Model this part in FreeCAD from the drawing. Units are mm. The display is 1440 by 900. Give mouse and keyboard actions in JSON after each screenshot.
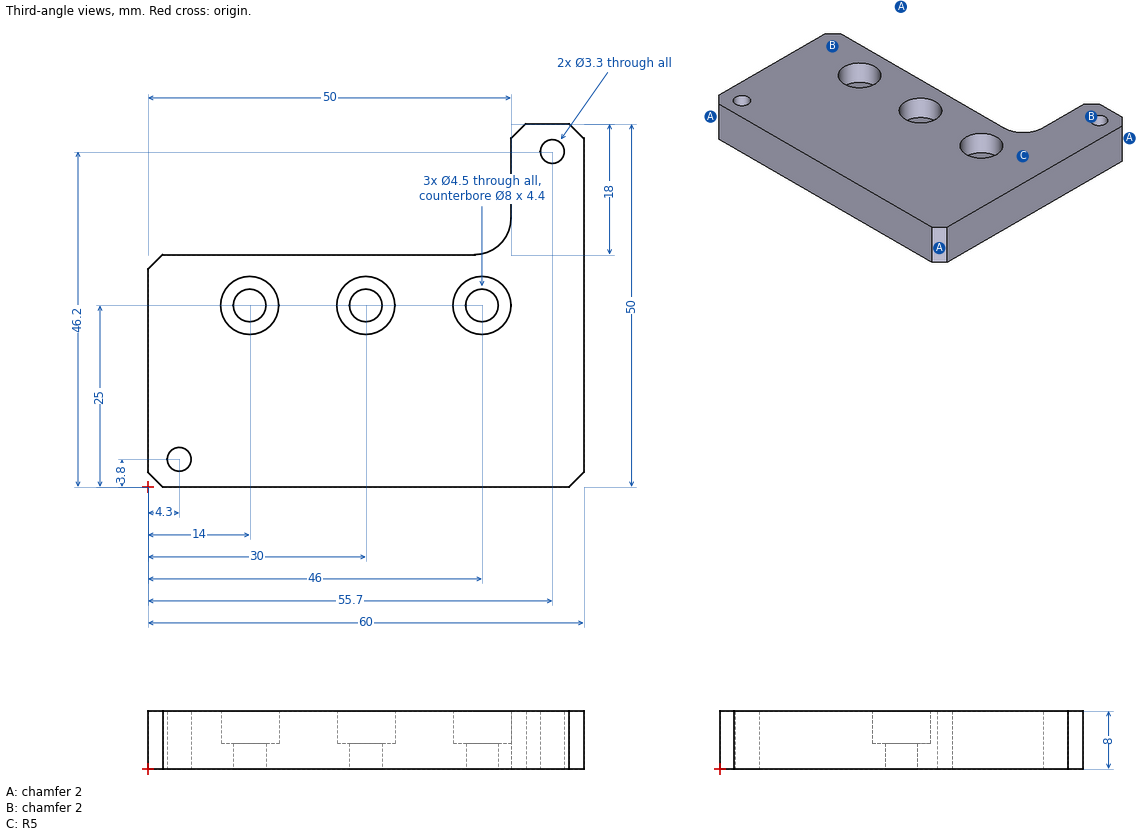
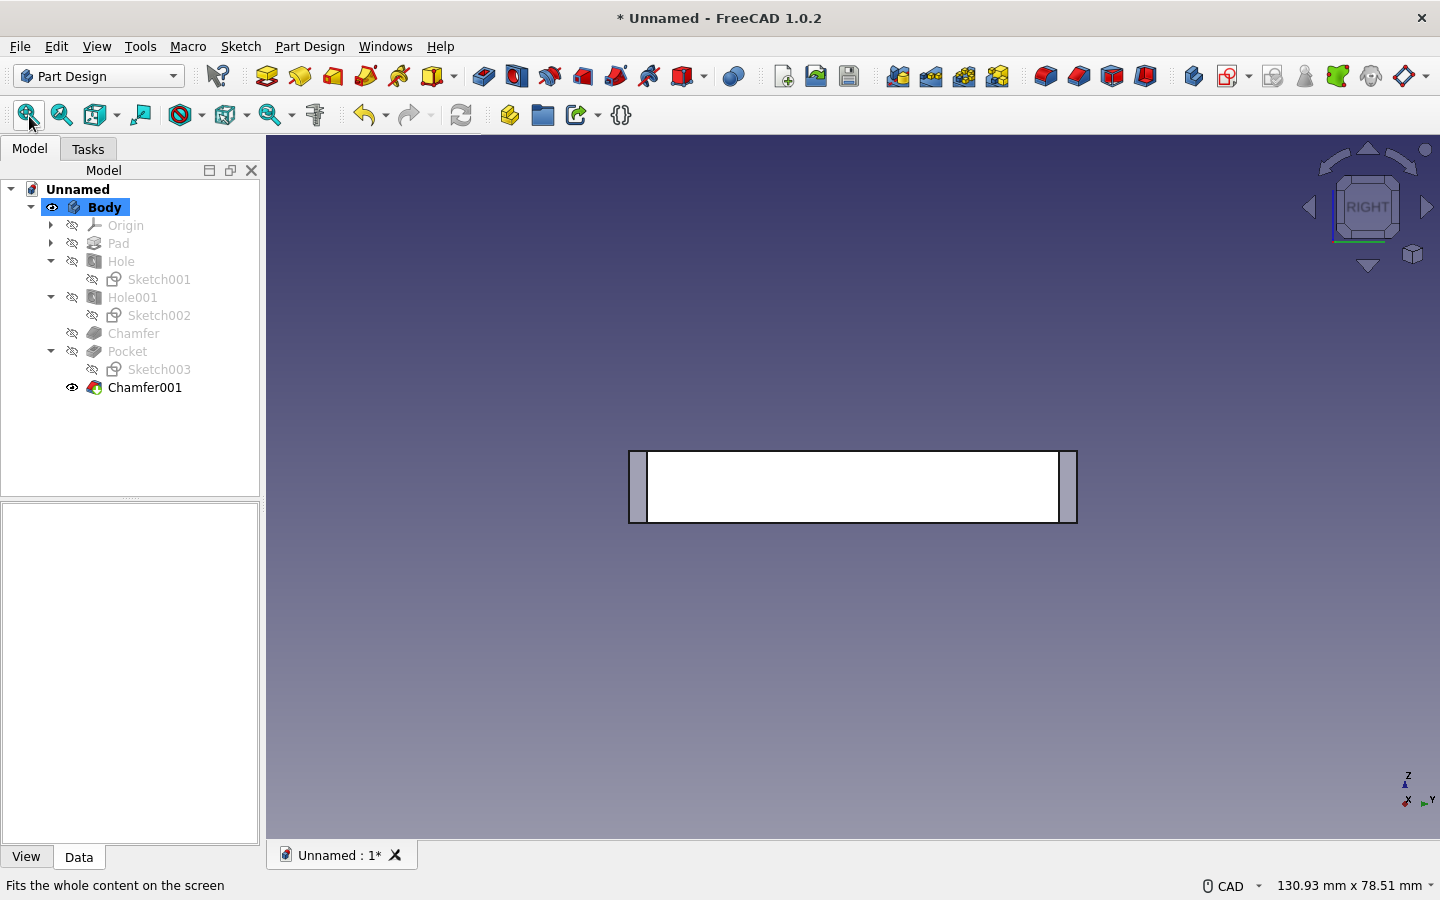
{"action": "key", "text": "5"}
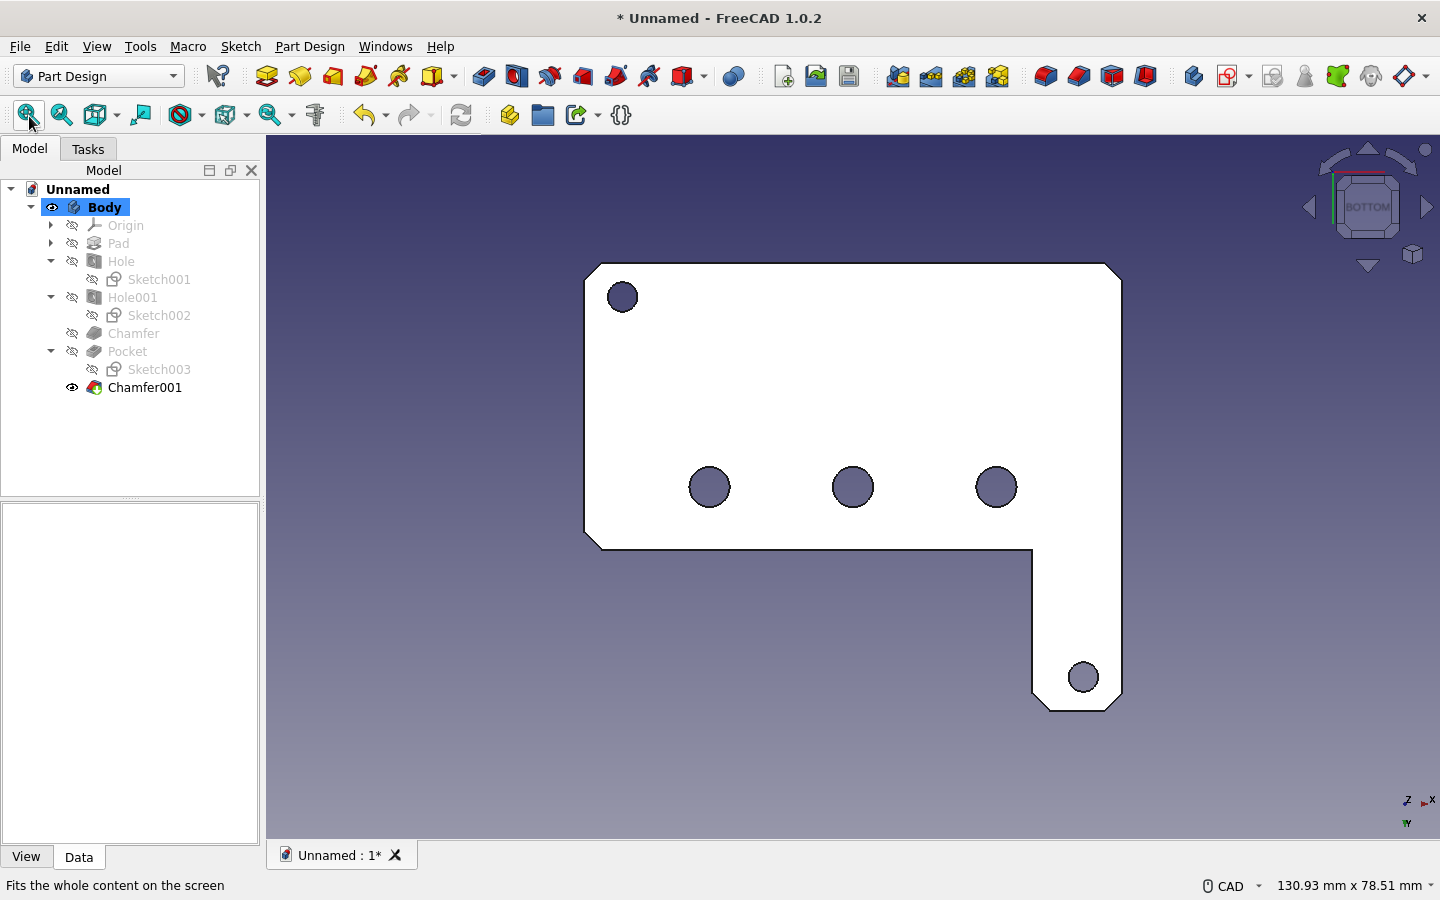
{"action": "key", "text": "4"}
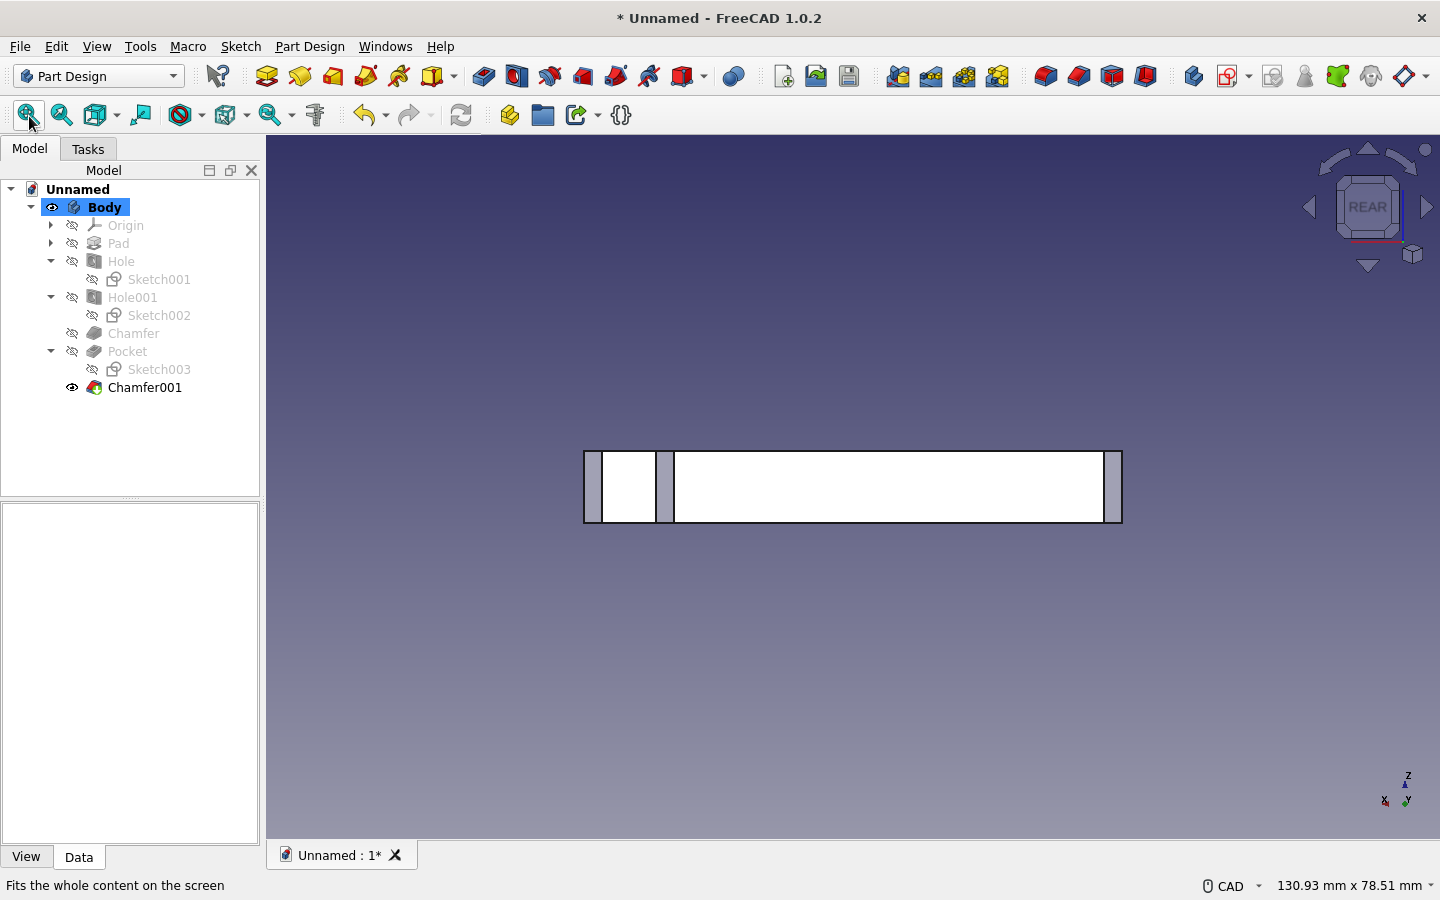
{"action": "key", "text": "6"}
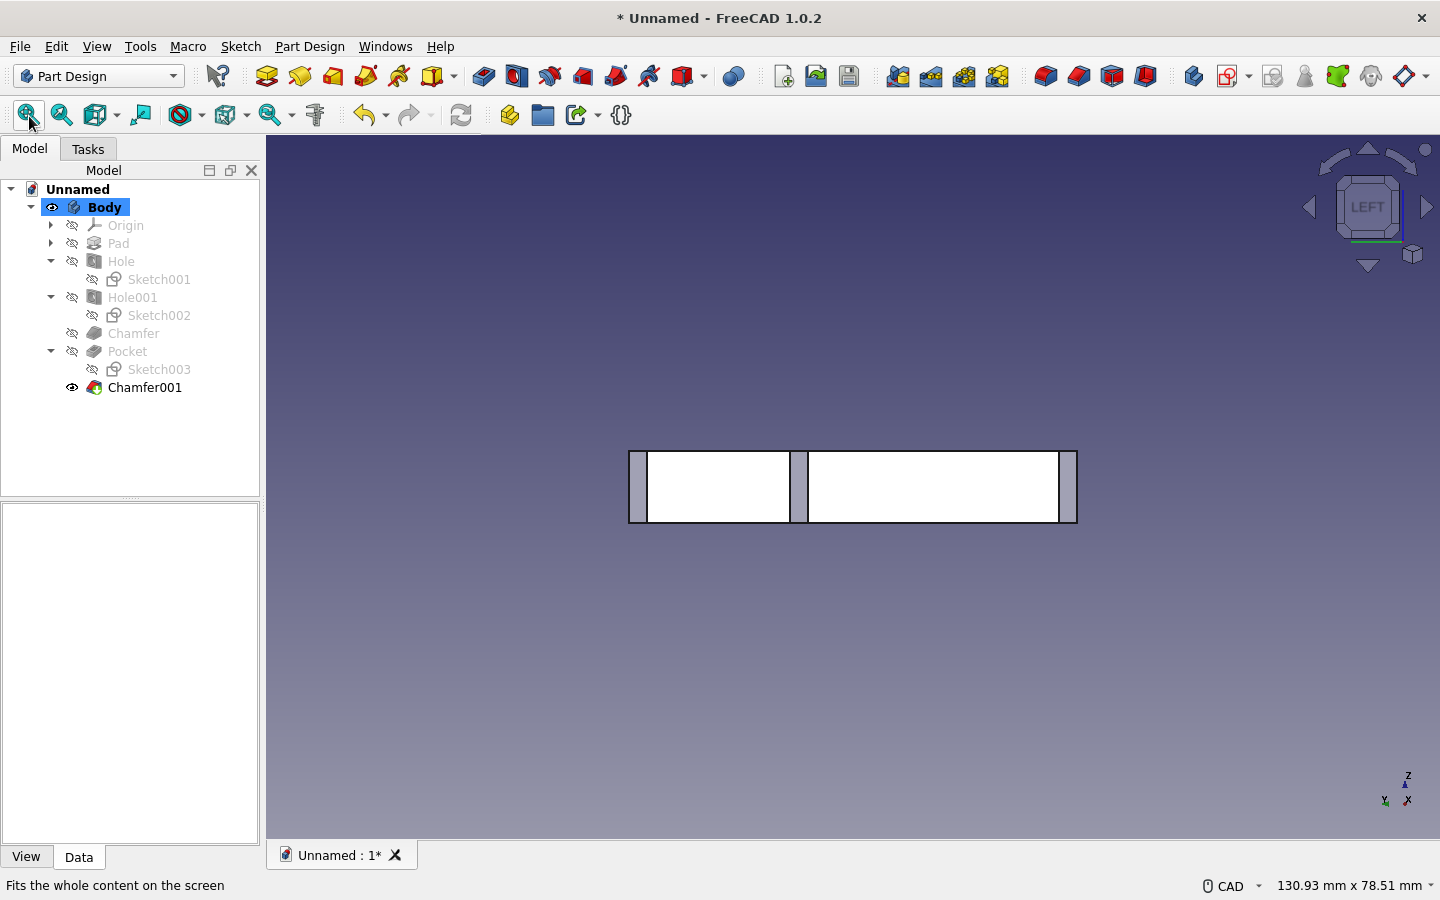
{"action": "left_click", "coordinate": [29, 116]}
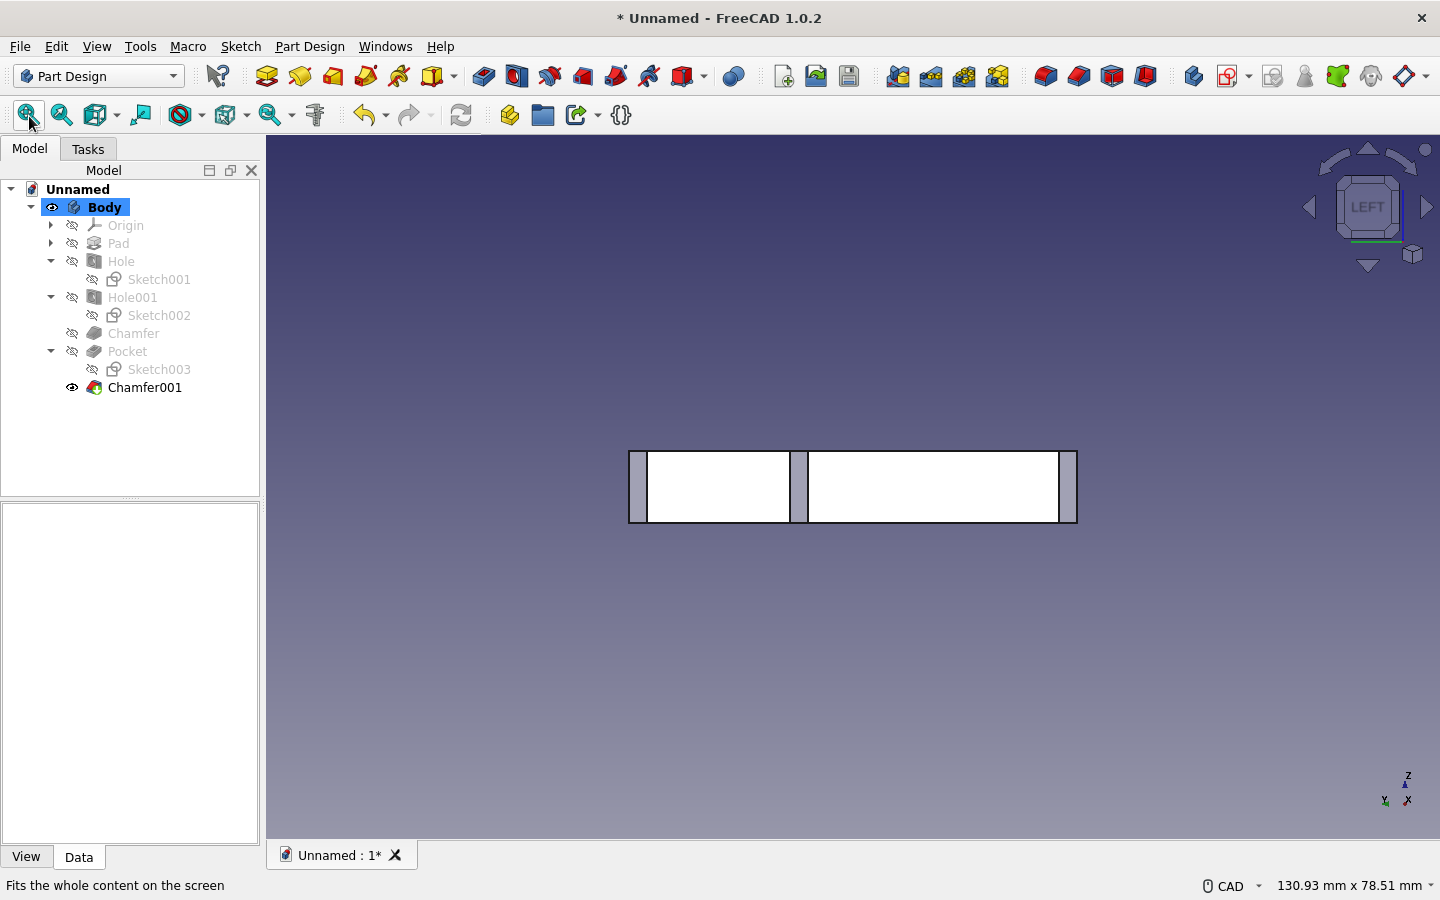
{"action": "key", "text": "v 3"}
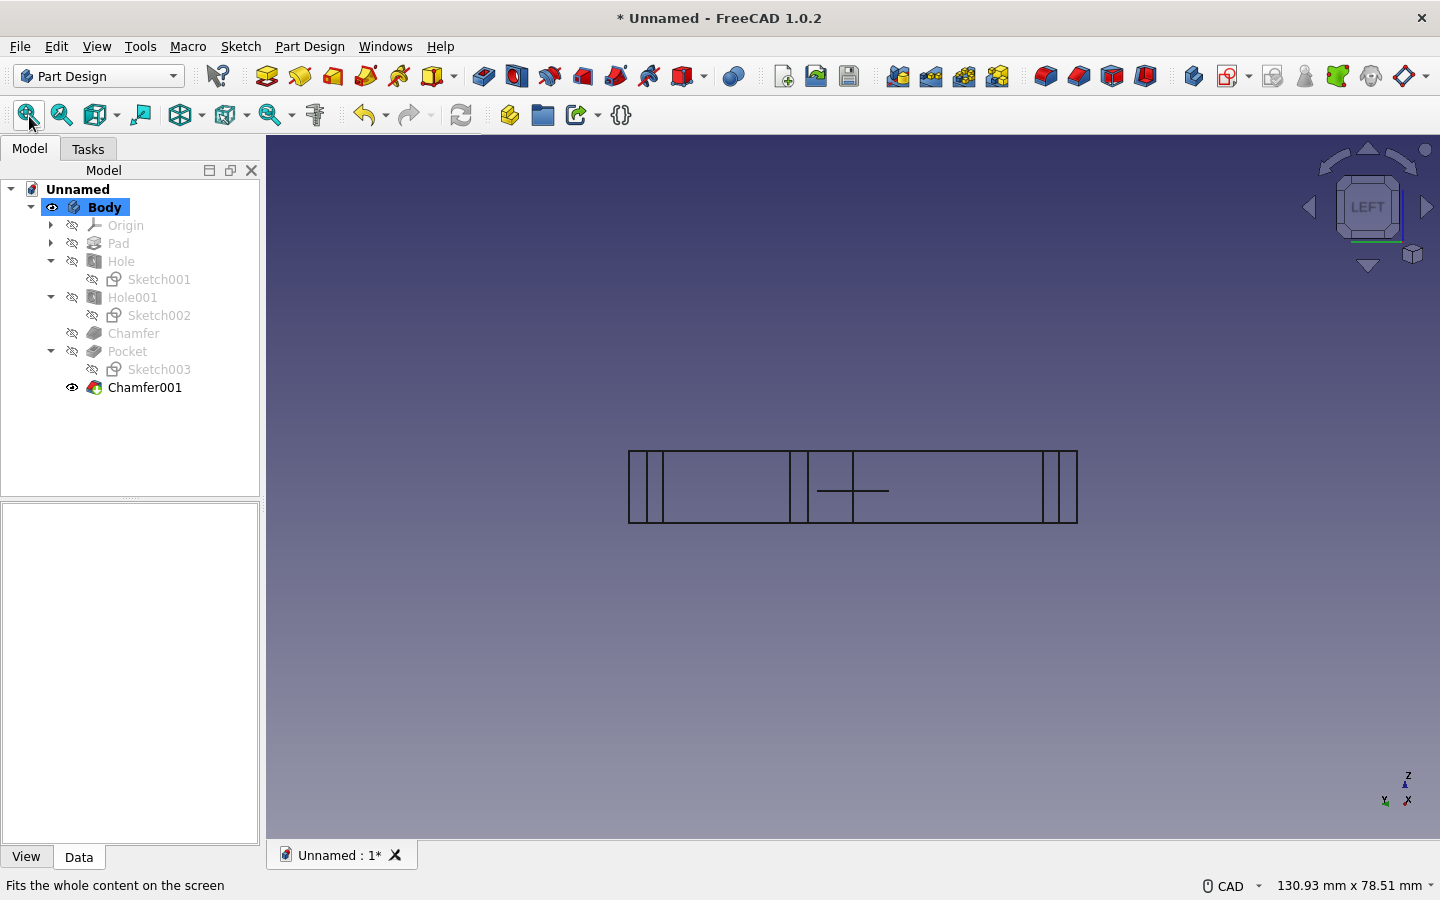
{"action": "key", "text": "0"}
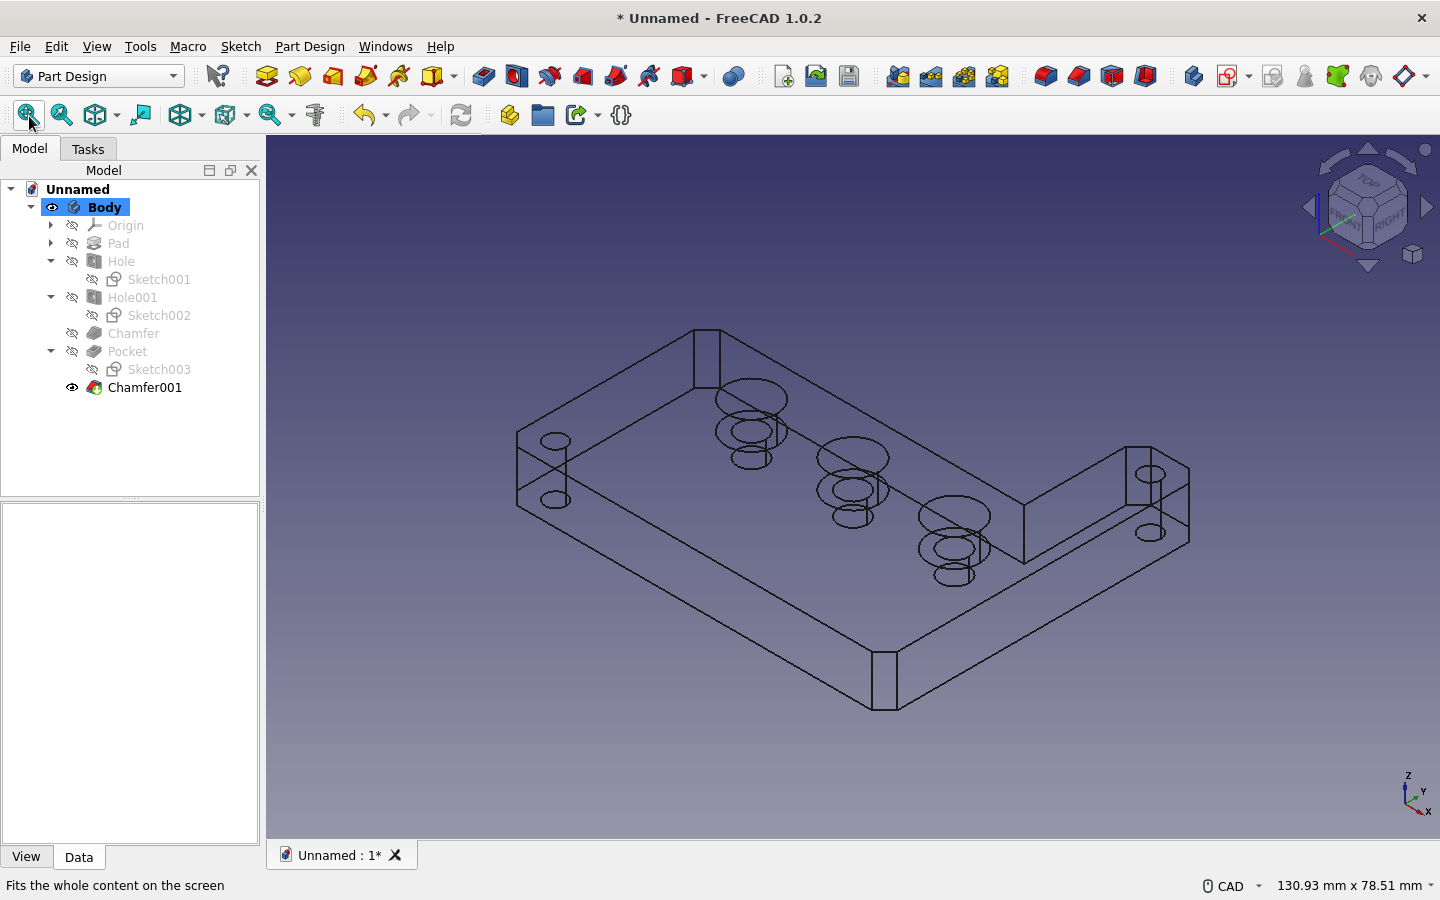
{"action": "left_click", "coordinate": [1024, 534]}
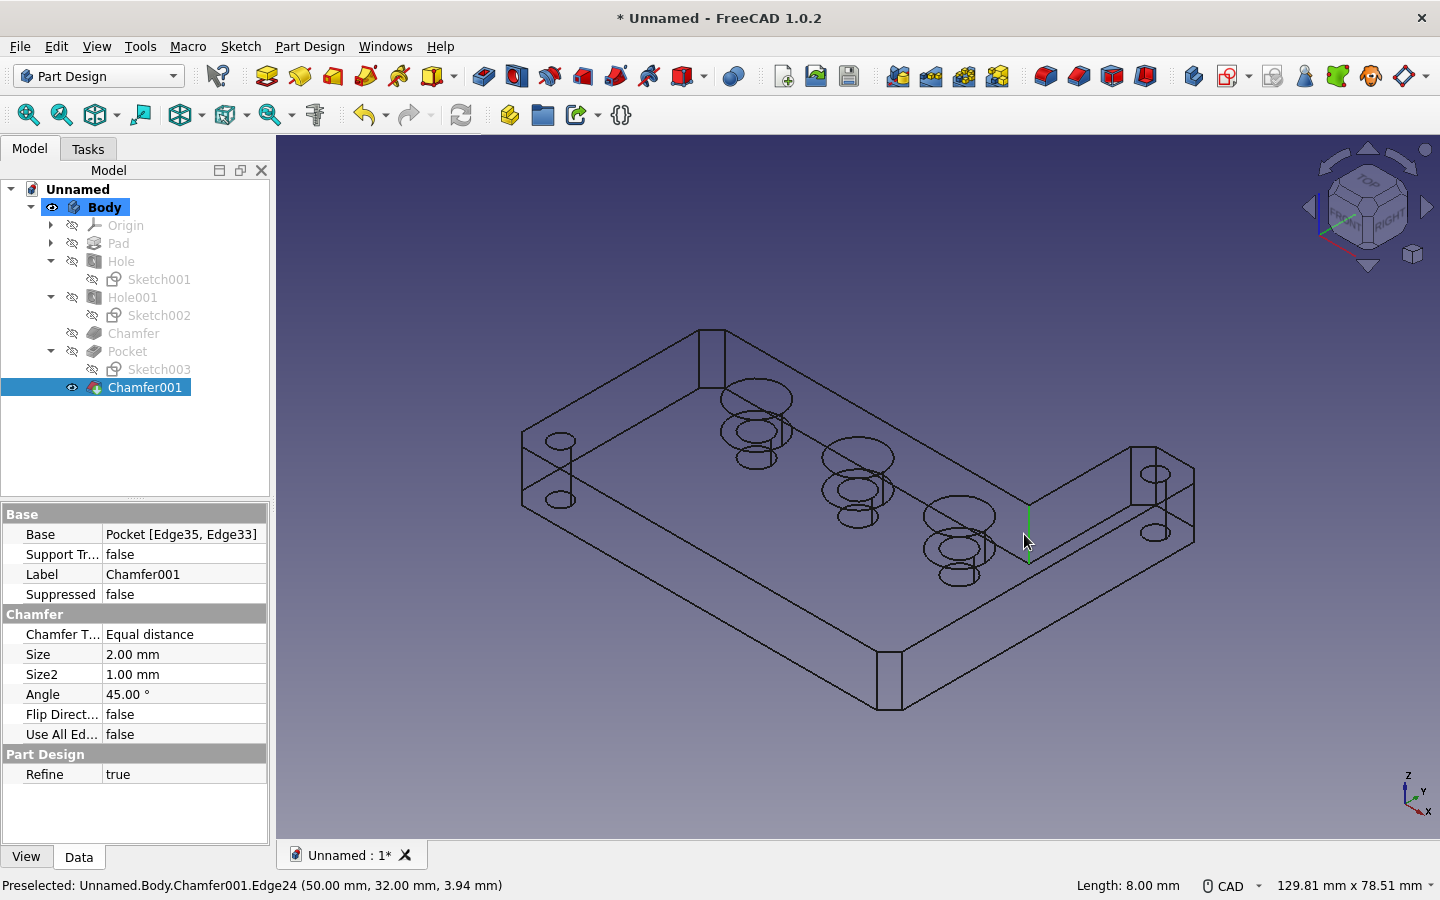
{"action": "key", "text": "v 1"}